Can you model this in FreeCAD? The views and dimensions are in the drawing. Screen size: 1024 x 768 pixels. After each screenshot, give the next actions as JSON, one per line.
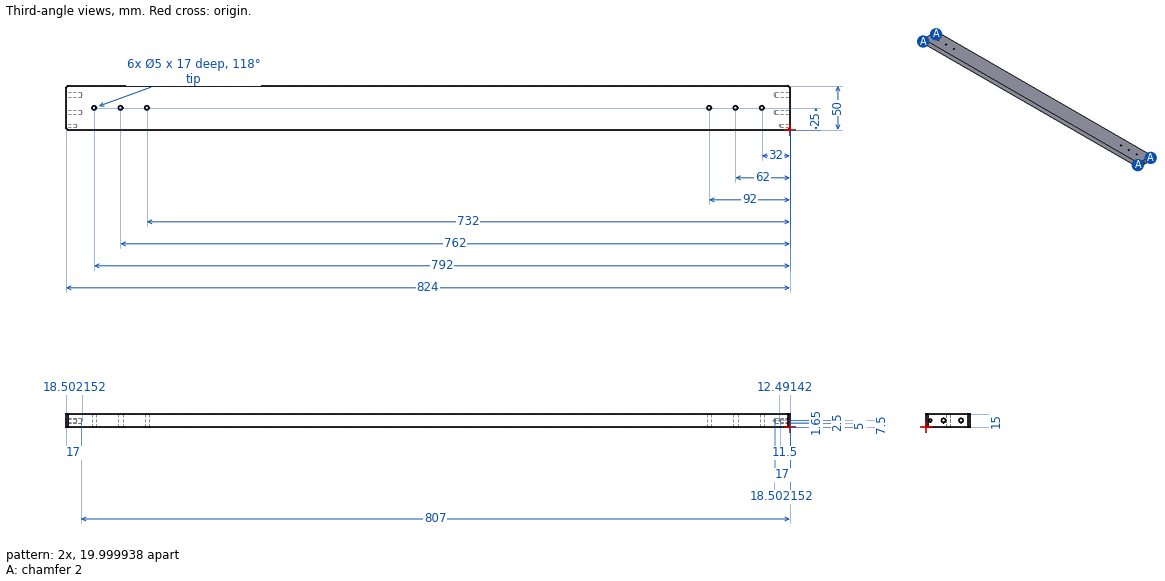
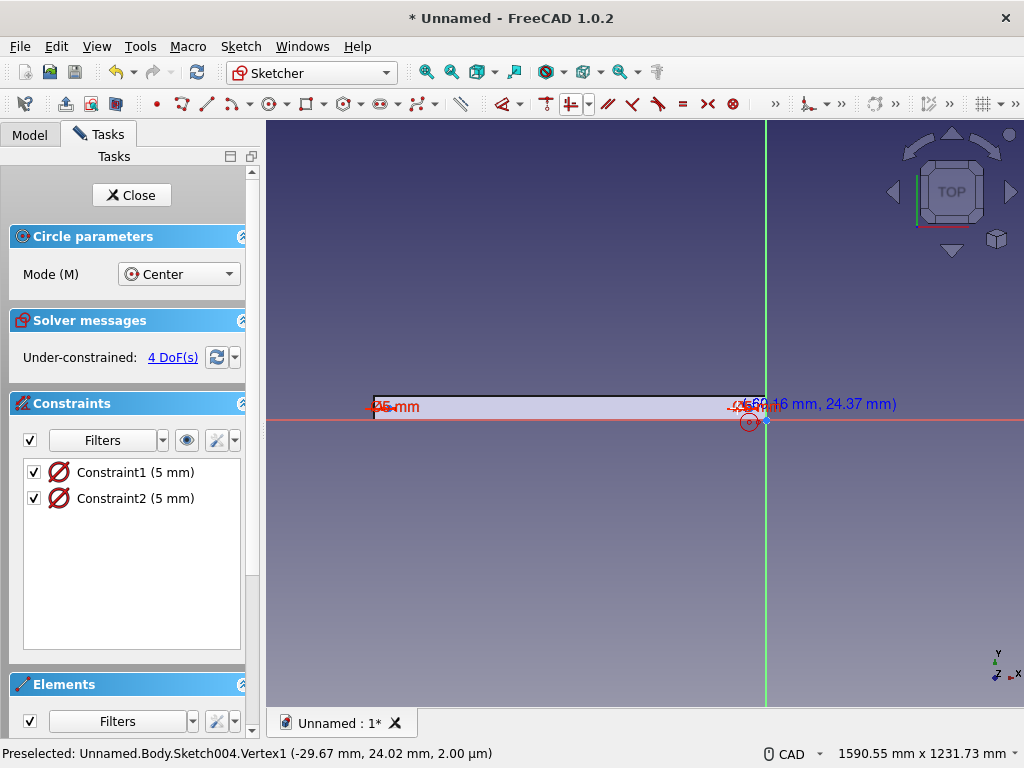
{"action": "scroll", "coordinate": [737, 408], "scroll_direction": "up", "scroll_amount": 2}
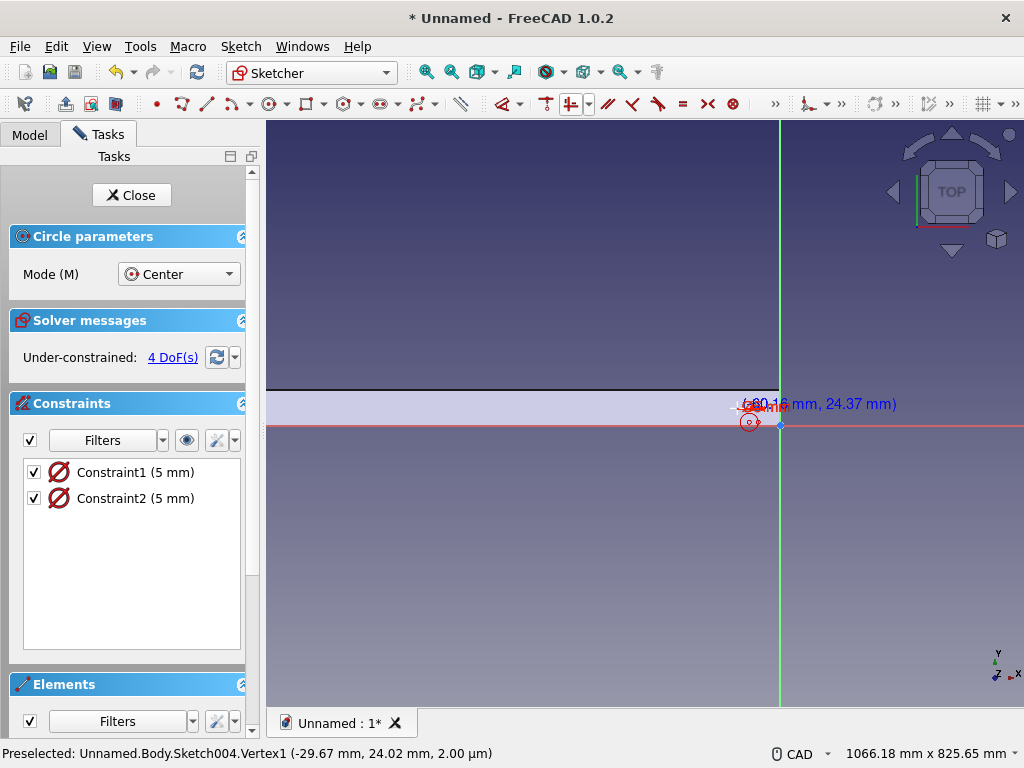
{"action": "left_click", "coordinate": [736, 408]}
{"action": "mouse_move", "coordinate": [738, 407]}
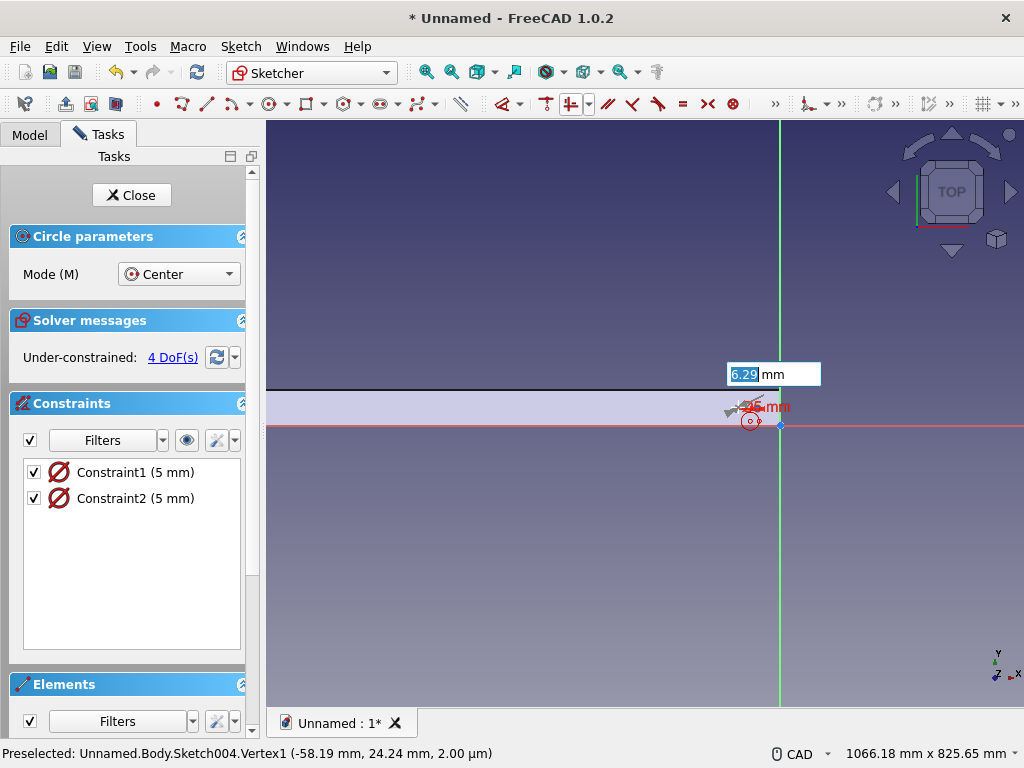
{"action": "type", "text": "5"}
{"action": "key", "text": "Return"}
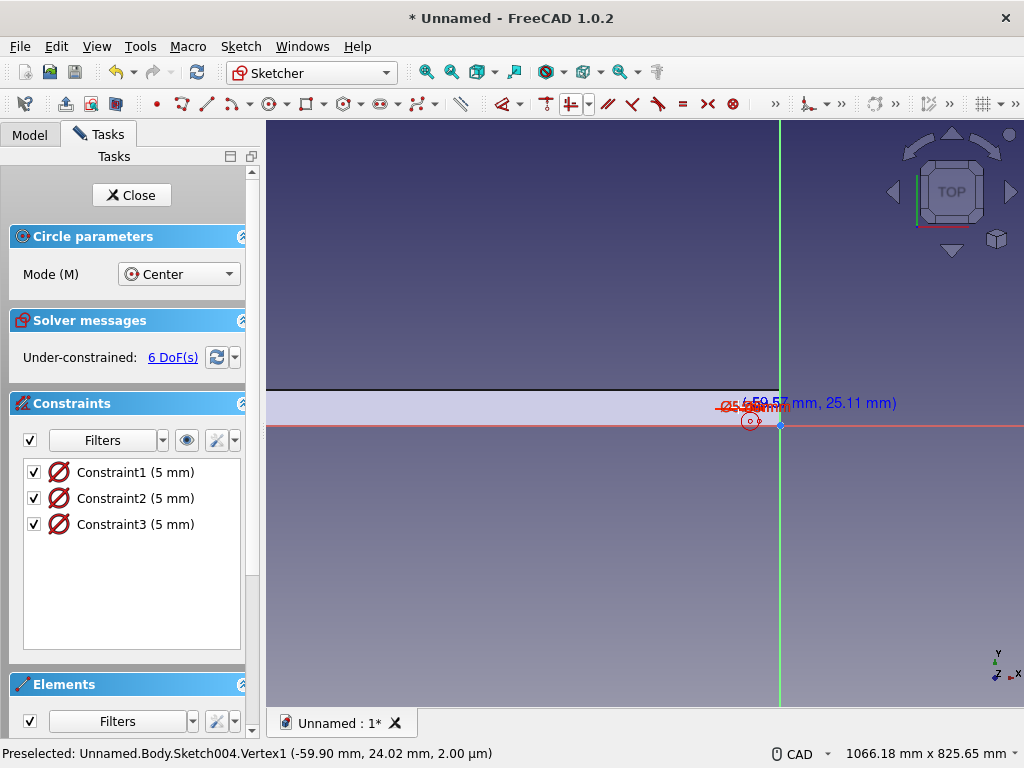
{"action": "scroll", "coordinate": [715, 408], "scroll_direction": "up", "scroll_amount": 13}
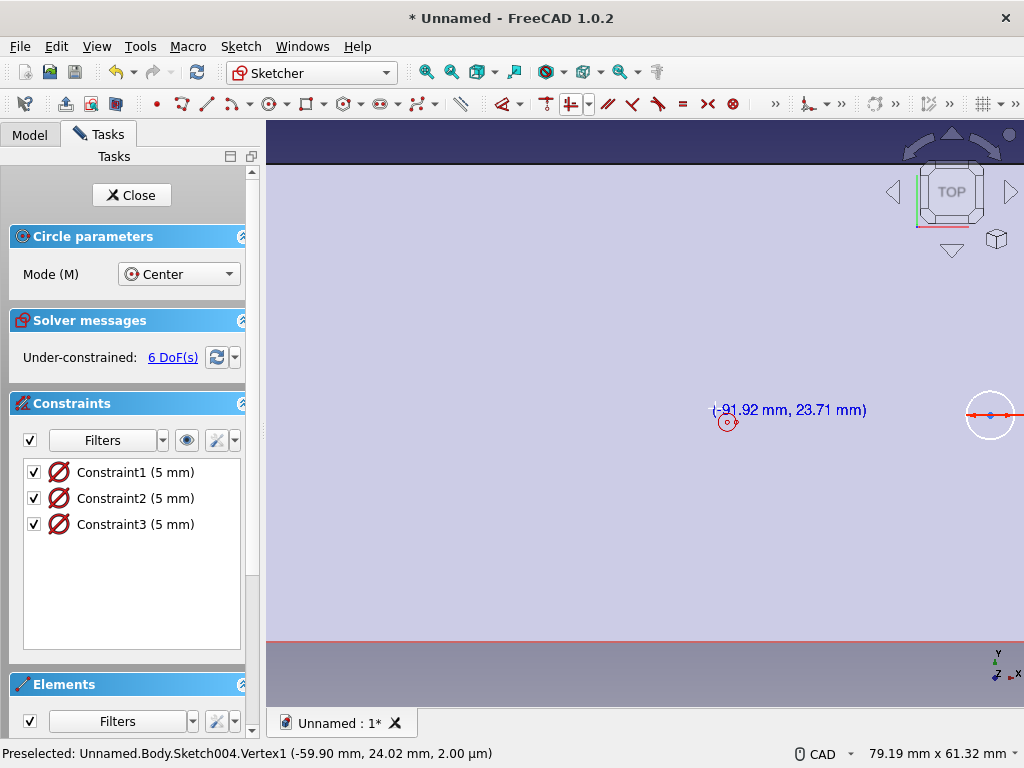
{"action": "scroll", "coordinate": [723, 408], "scroll_direction": "down", "scroll_amount": 15}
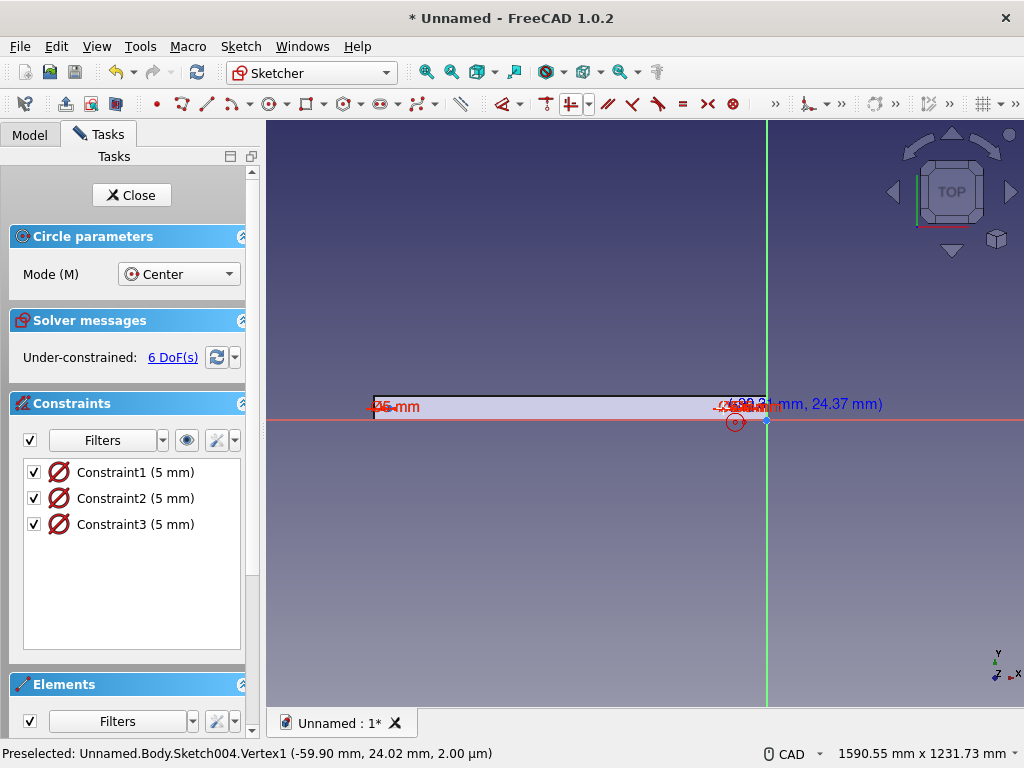
{"action": "scroll", "coordinate": [723, 408], "scroll_direction": "up", "scroll_amount": 2}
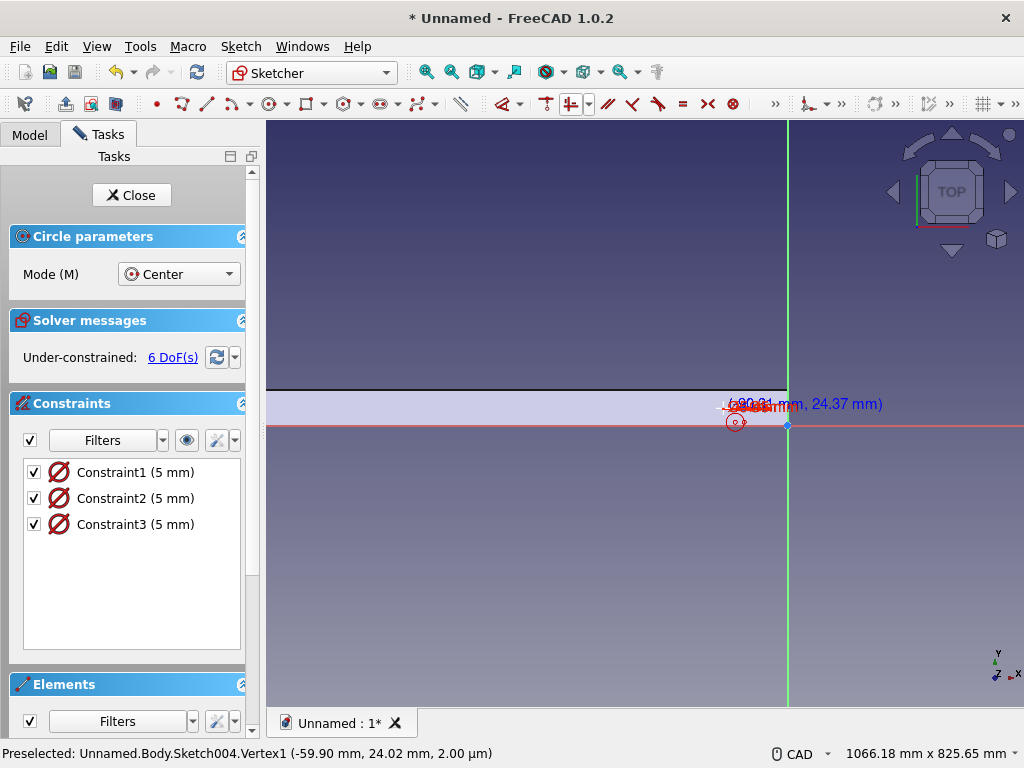
{"action": "left_click", "coordinate": [722, 408]}
{"action": "mouse_move", "coordinate": [724, 407]}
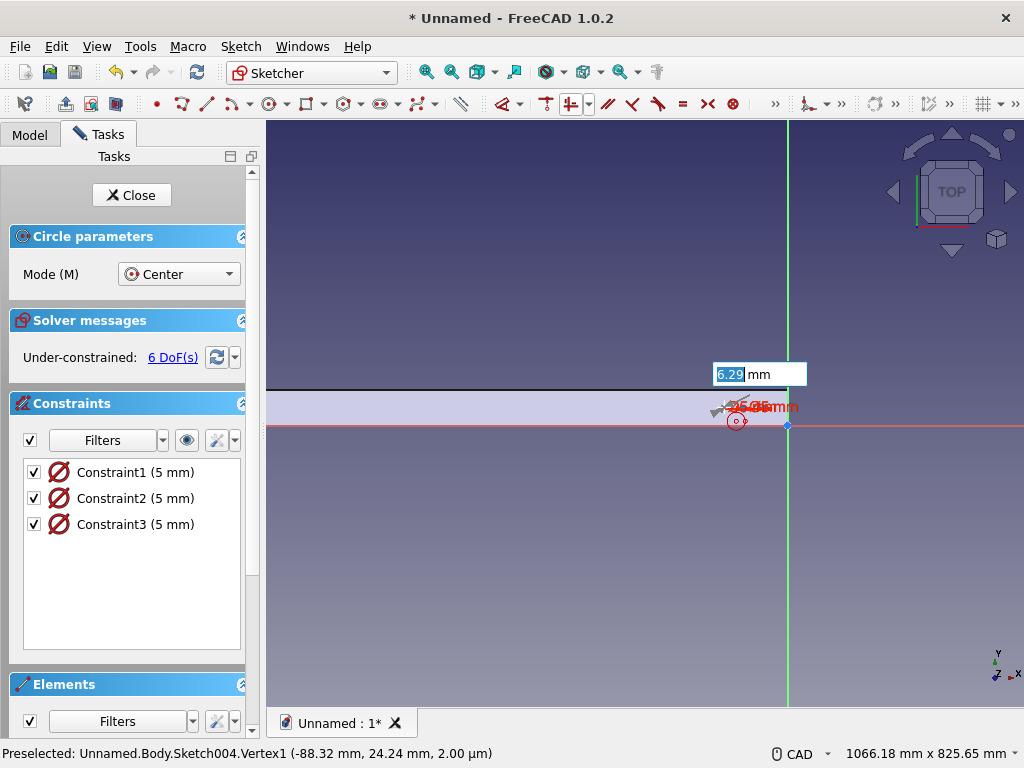
{"action": "type", "text": "5"}
{"action": "key", "text": "Return"}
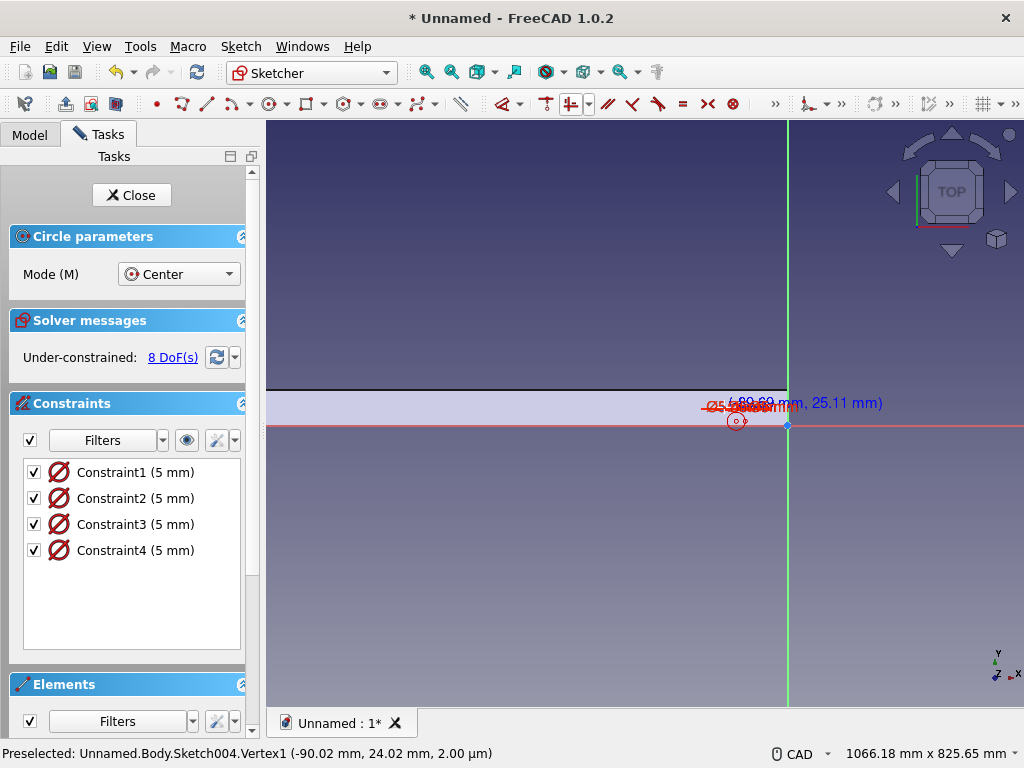
{"action": "scroll", "coordinate": [721, 408], "scroll_direction": "down", "scroll_amount": 2}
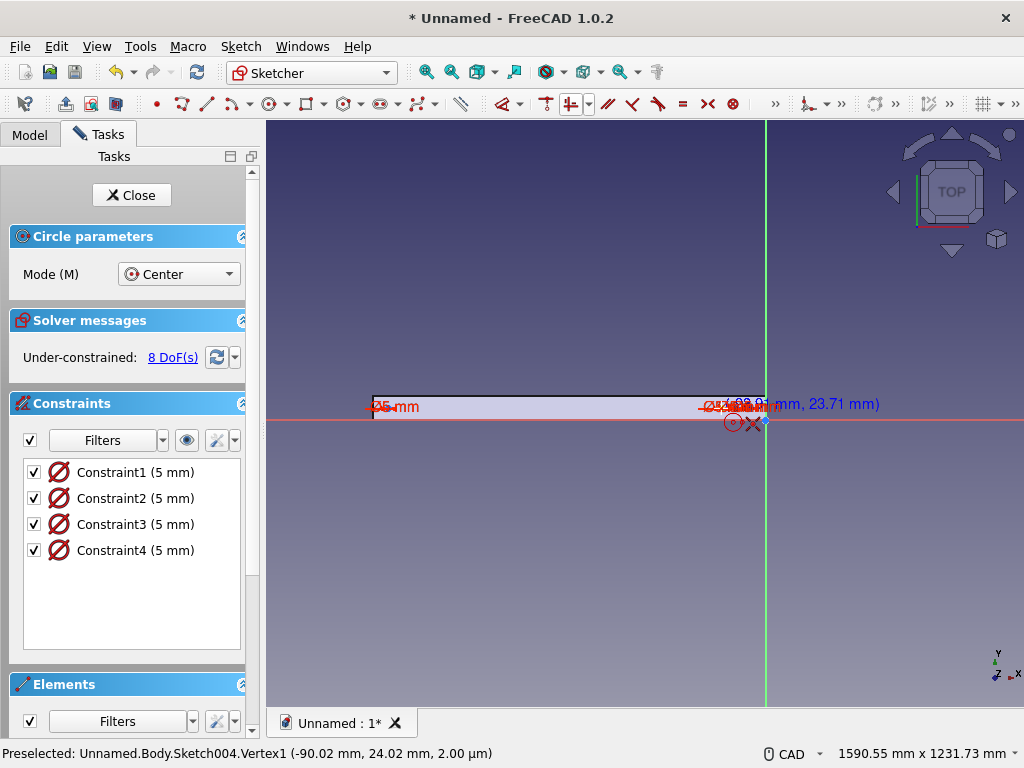
{"action": "scroll", "coordinate": [417, 408], "scroll_direction": "up", "scroll_amount": 15}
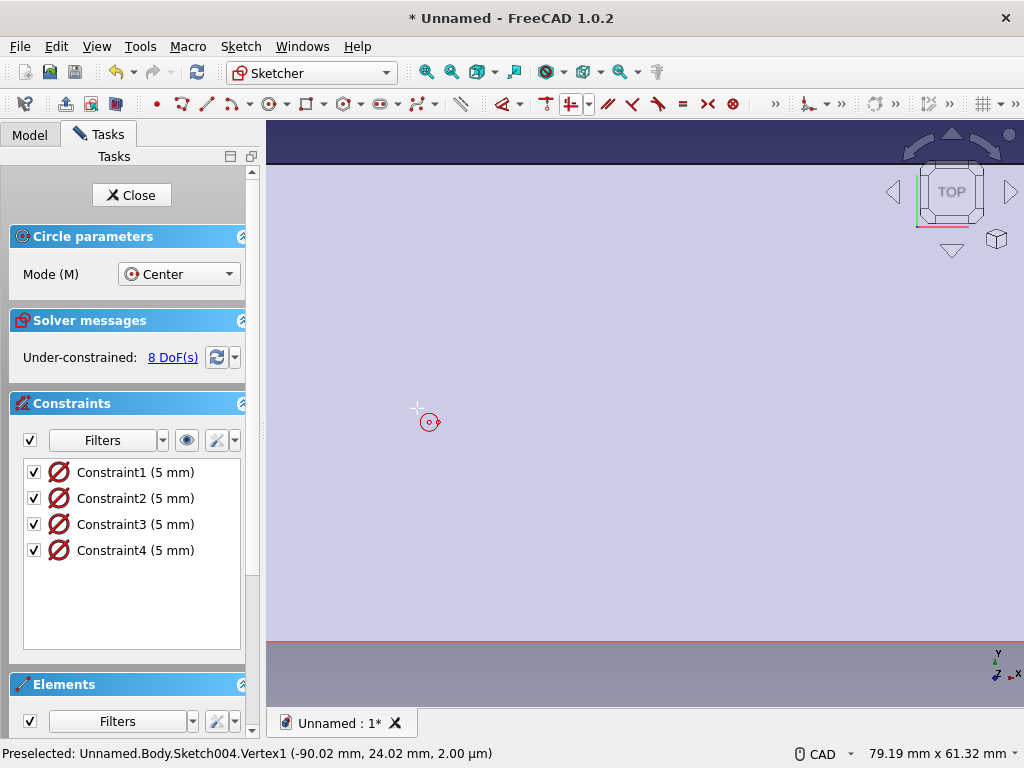
{"action": "scroll", "coordinate": [417, 408], "scroll_direction": "down", "scroll_amount": 15}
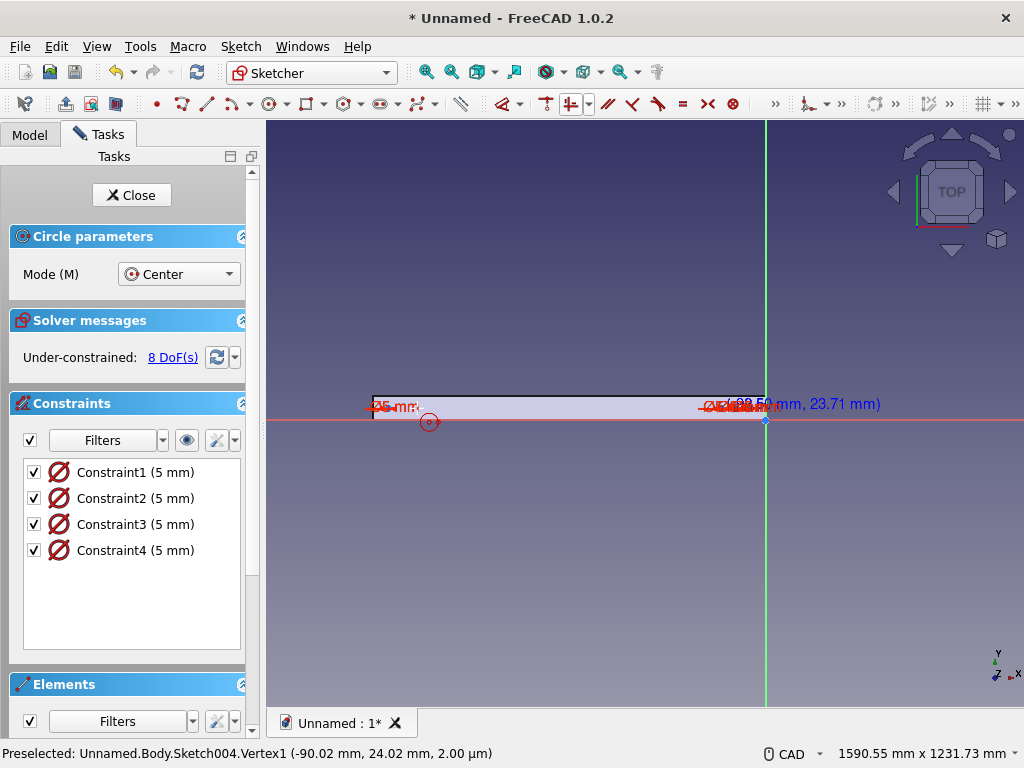
{"action": "scroll", "coordinate": [417, 408], "scroll_direction": "up", "scroll_amount": 2}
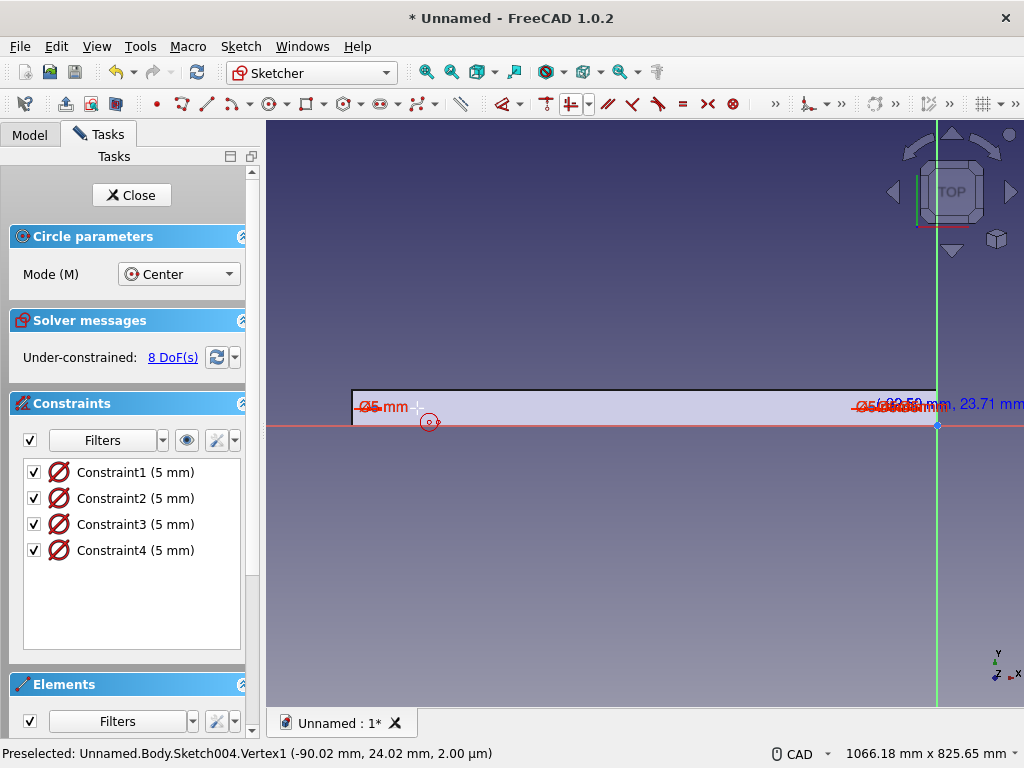
{"action": "left_click", "coordinate": [417, 408]}
{"action": "mouse_move", "coordinate": [418, 407]}